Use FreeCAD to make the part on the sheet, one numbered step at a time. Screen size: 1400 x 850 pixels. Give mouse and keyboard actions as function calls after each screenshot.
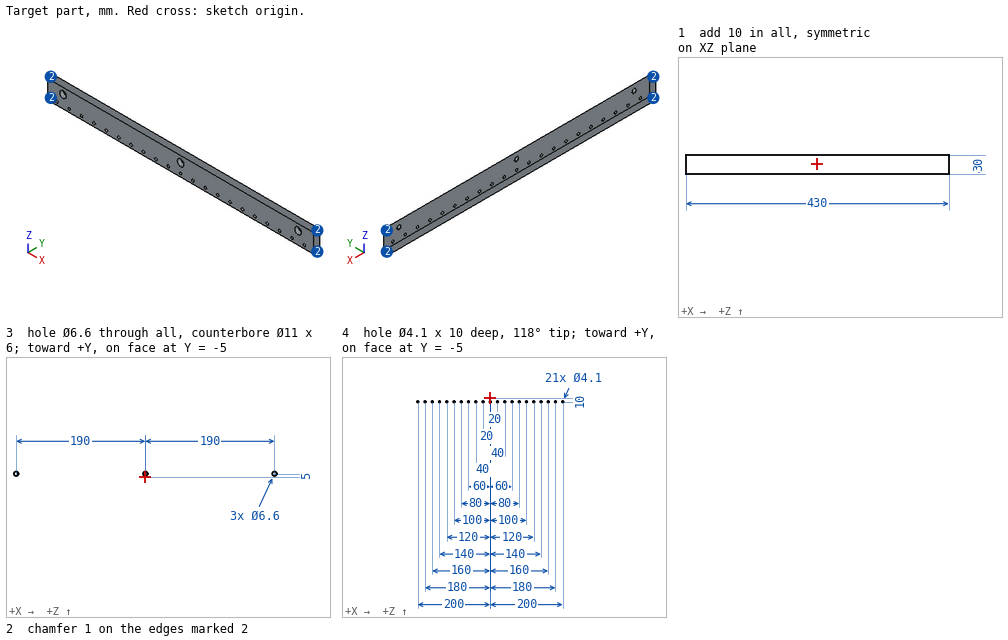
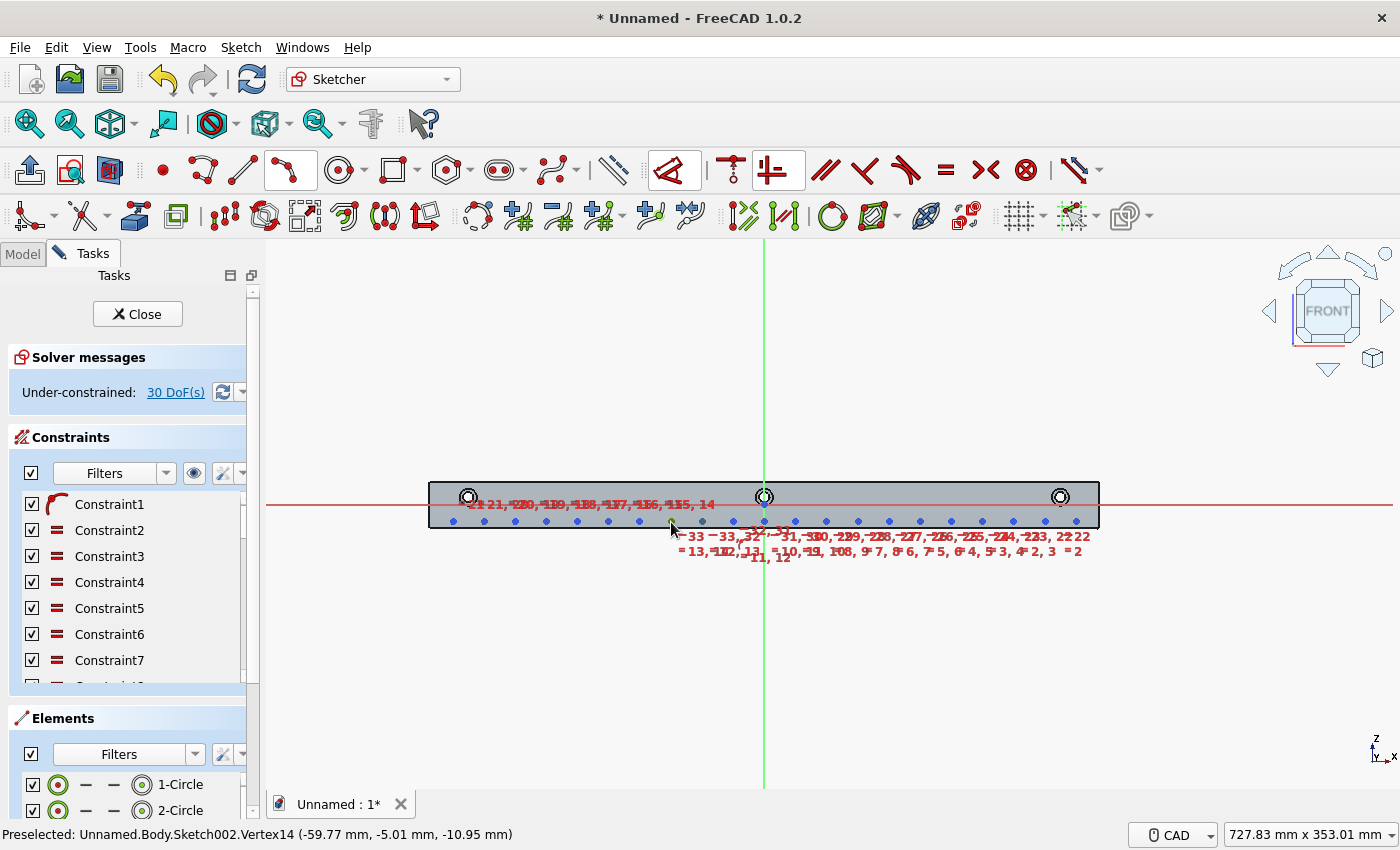
click(800, 170)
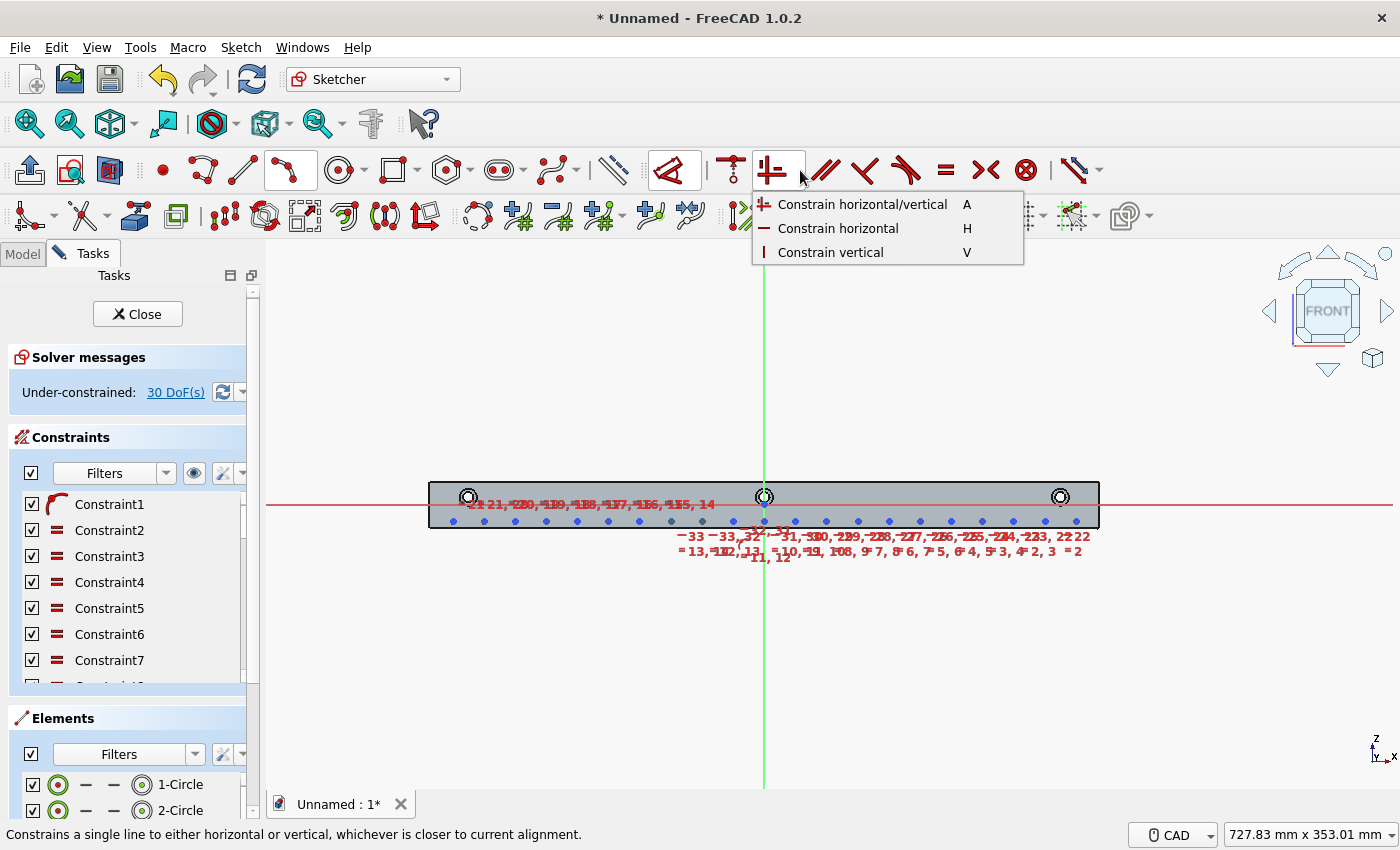
click(888, 228)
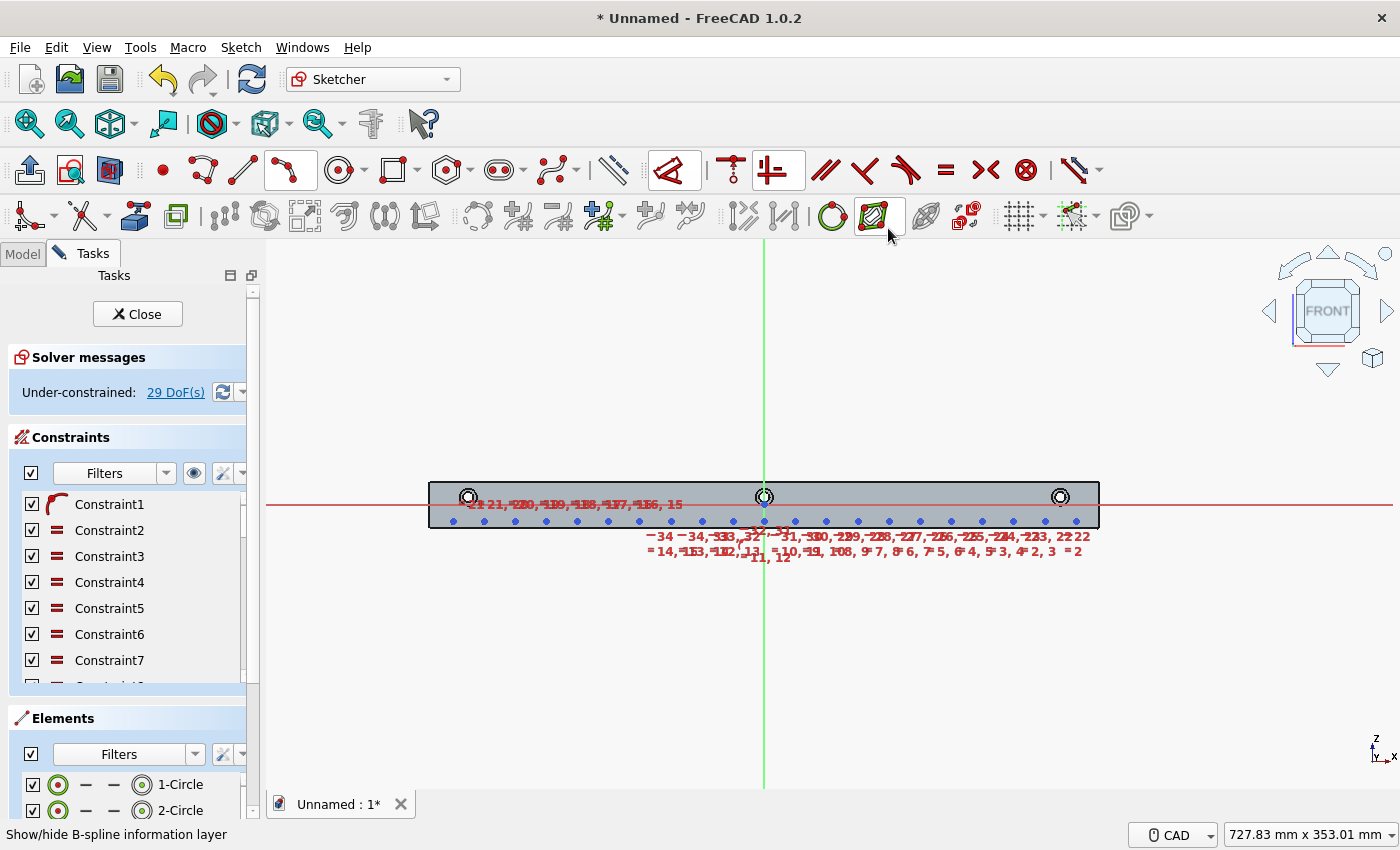
click(671, 522)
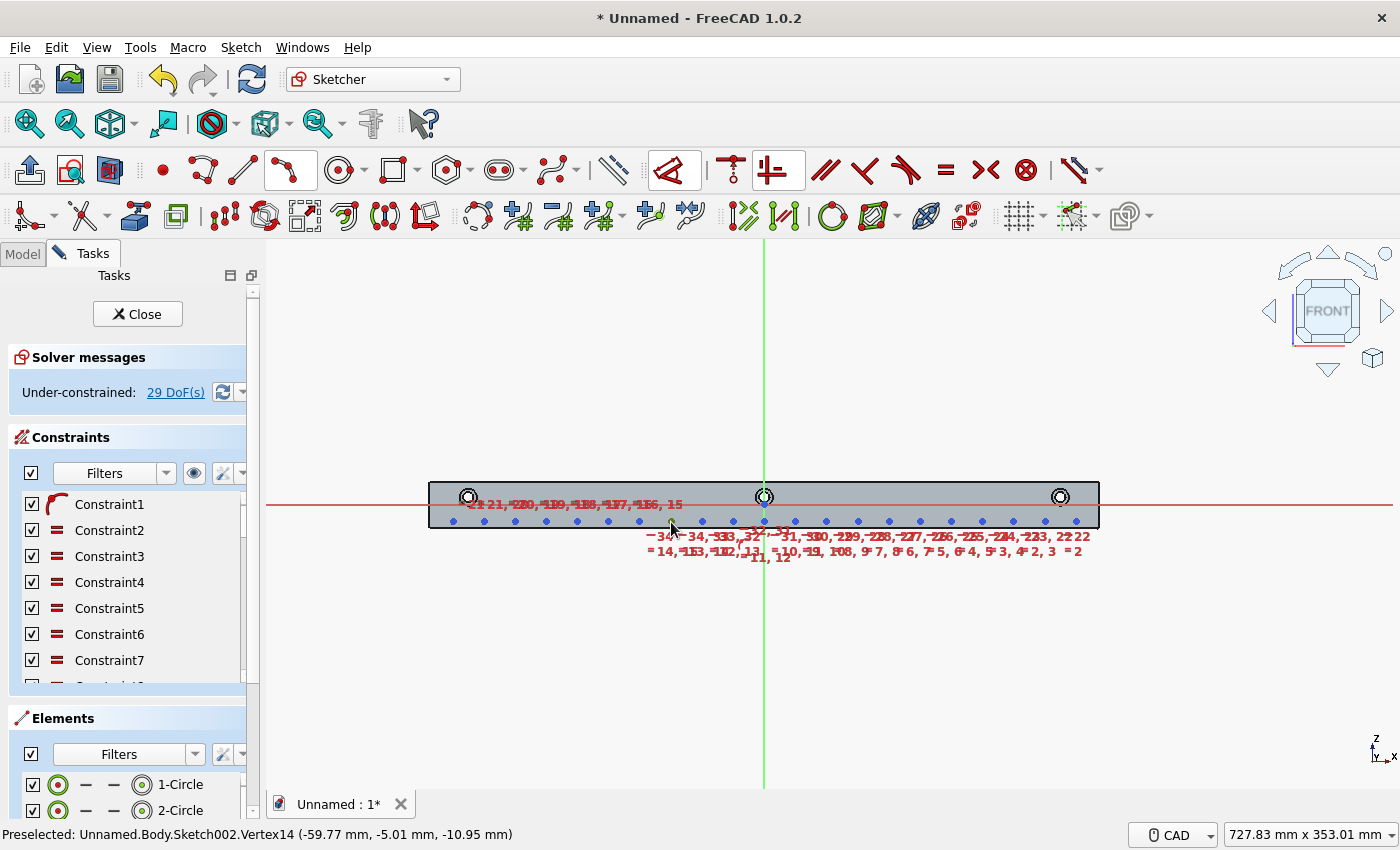
click(639, 522)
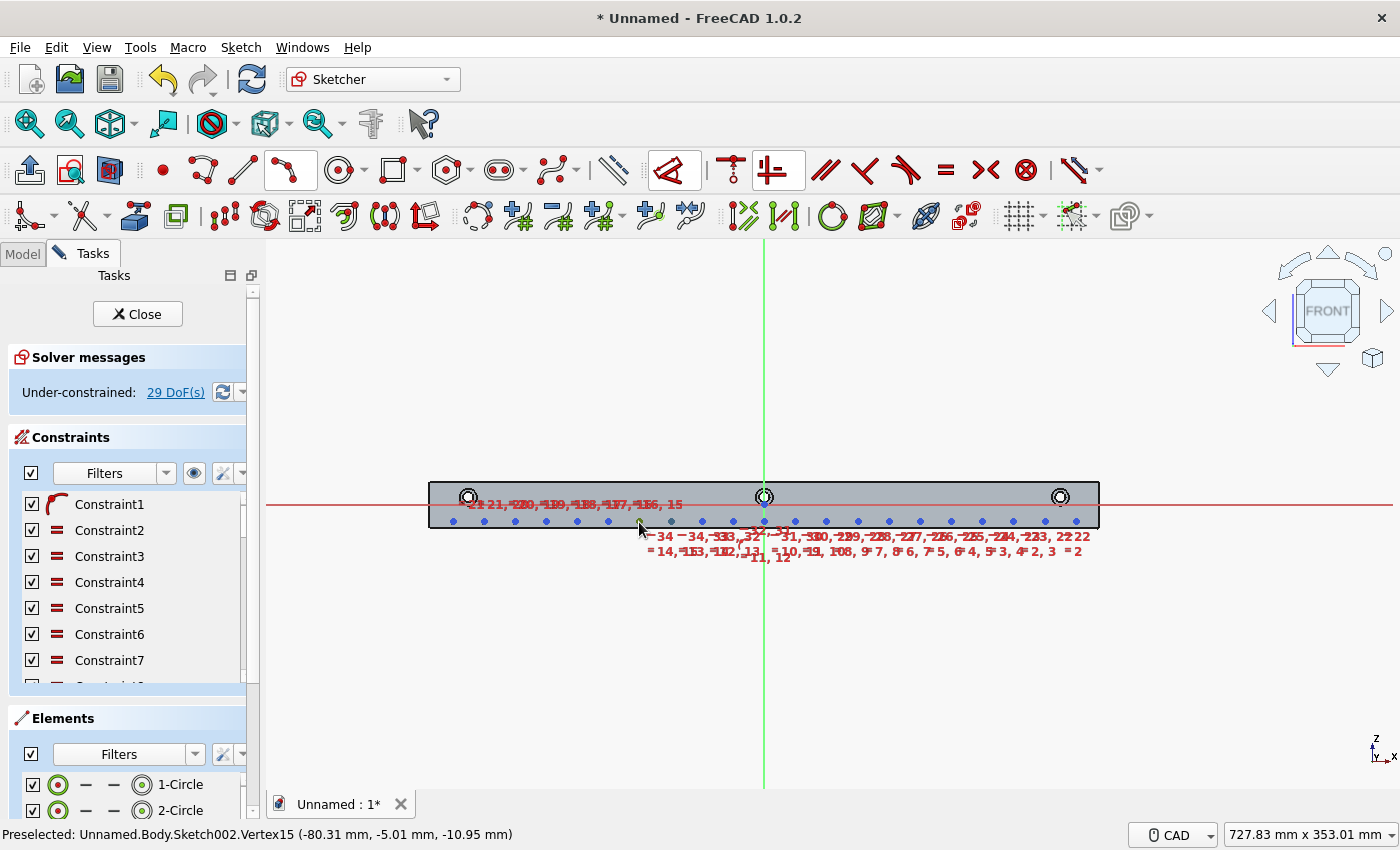
click(800, 170)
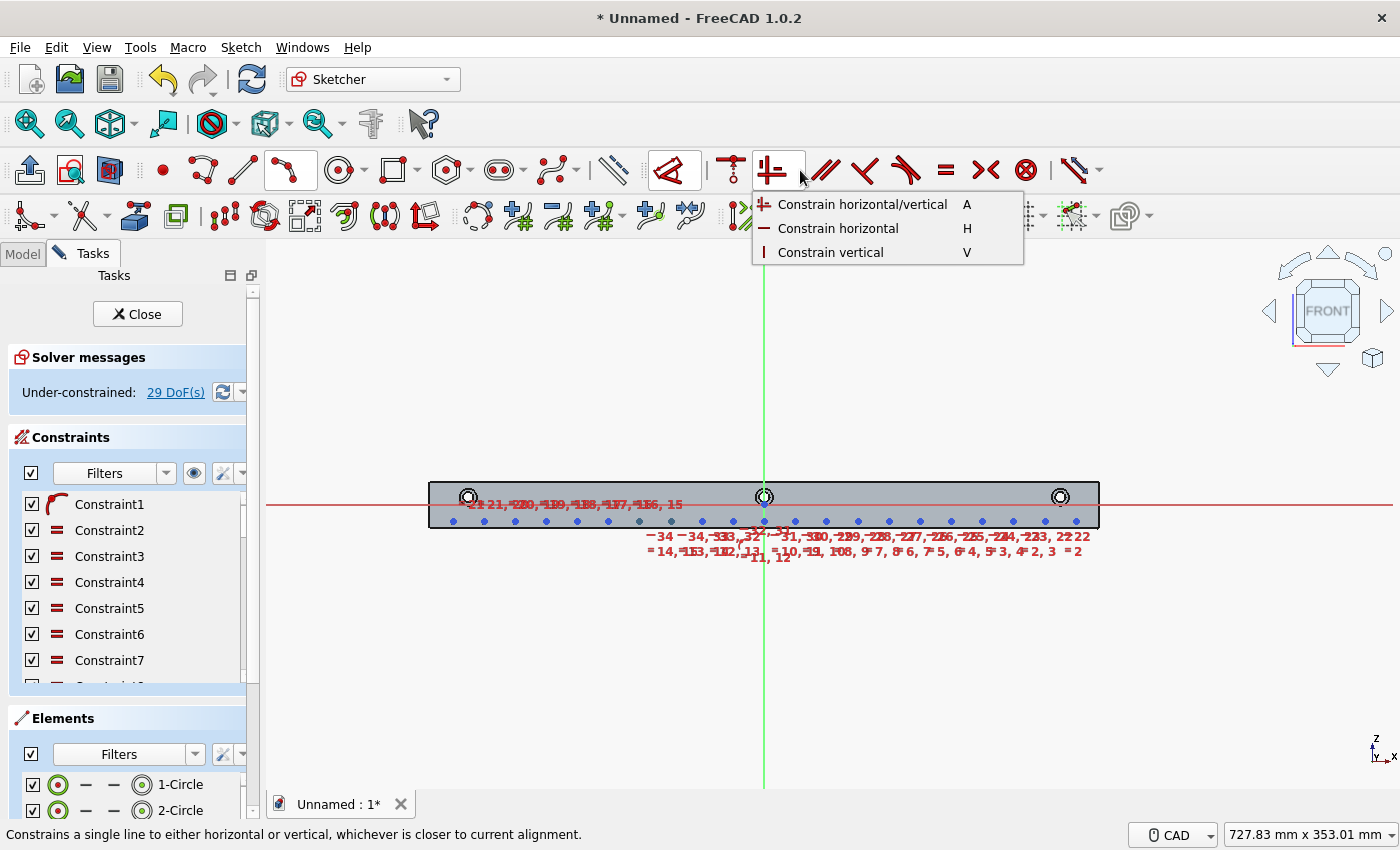
click(888, 228)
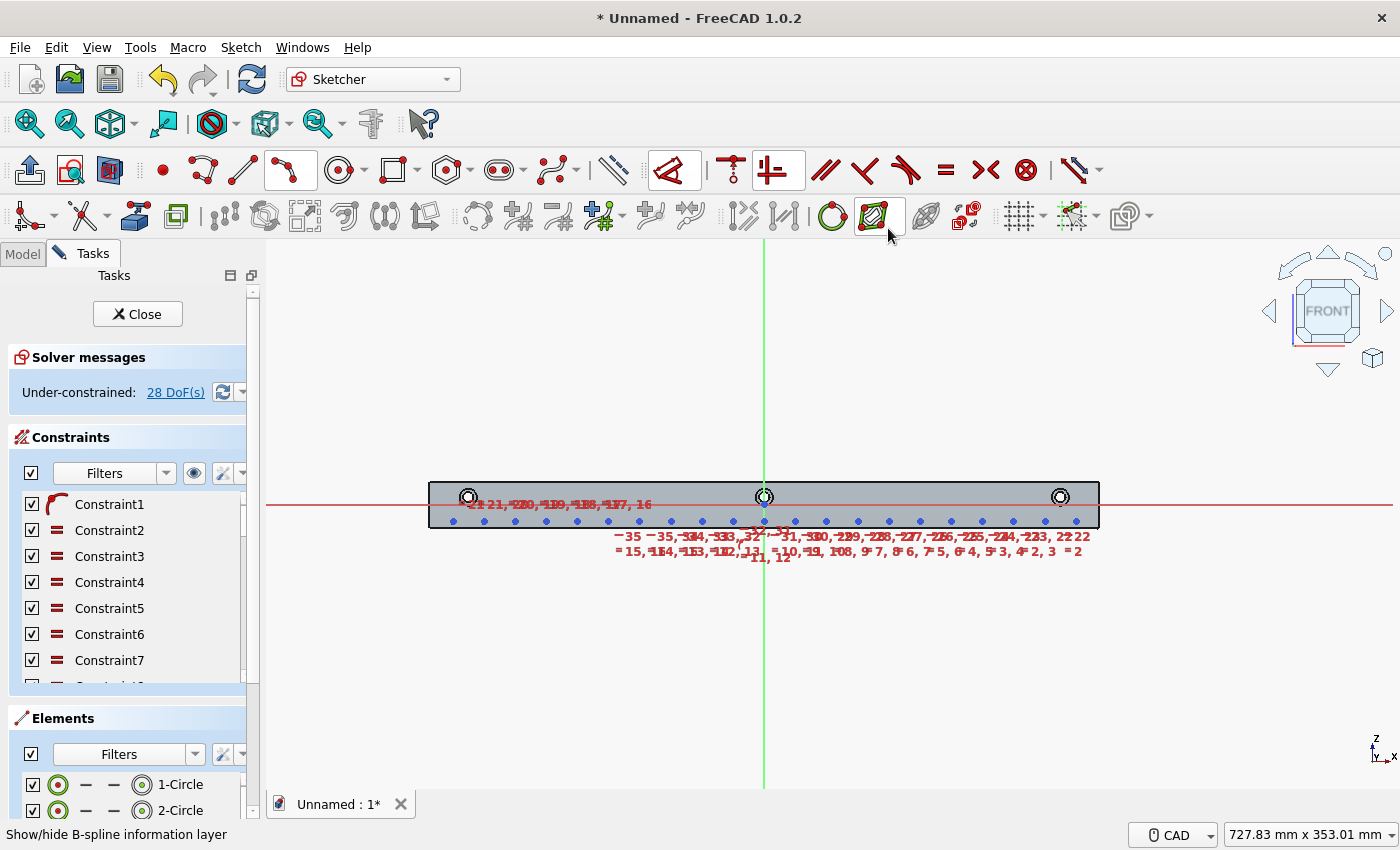
click(639, 522)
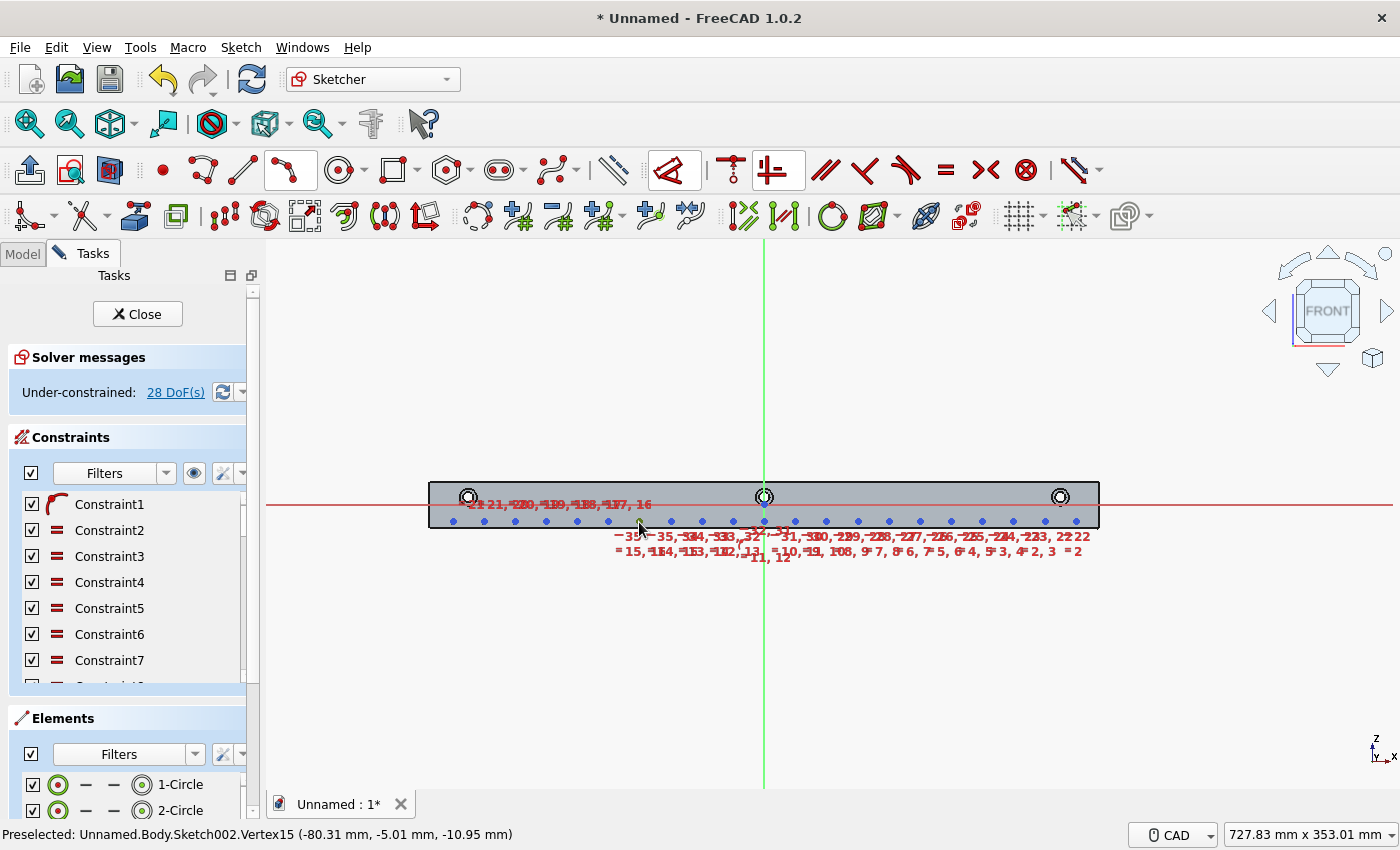
click(608, 522)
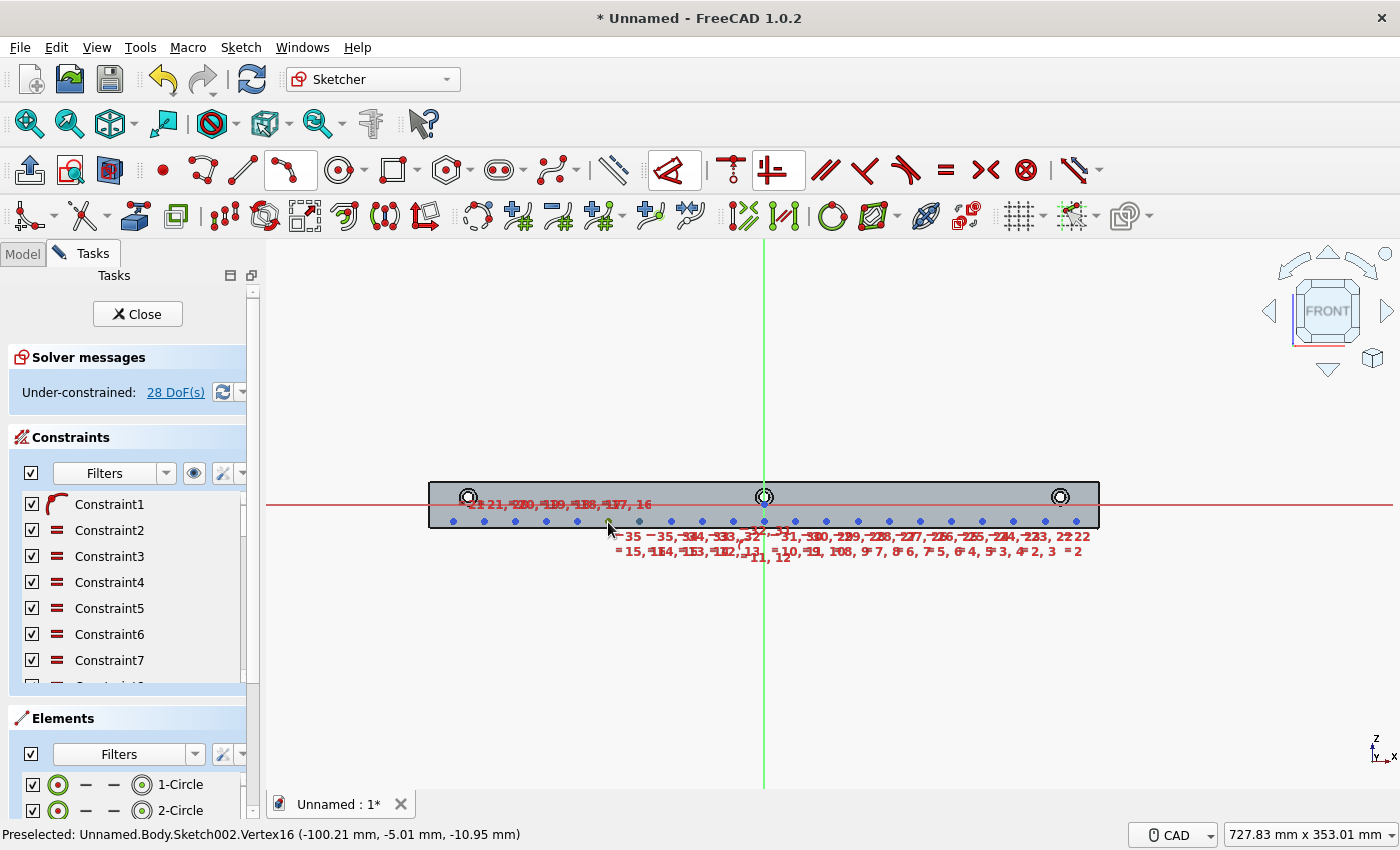
key(h)